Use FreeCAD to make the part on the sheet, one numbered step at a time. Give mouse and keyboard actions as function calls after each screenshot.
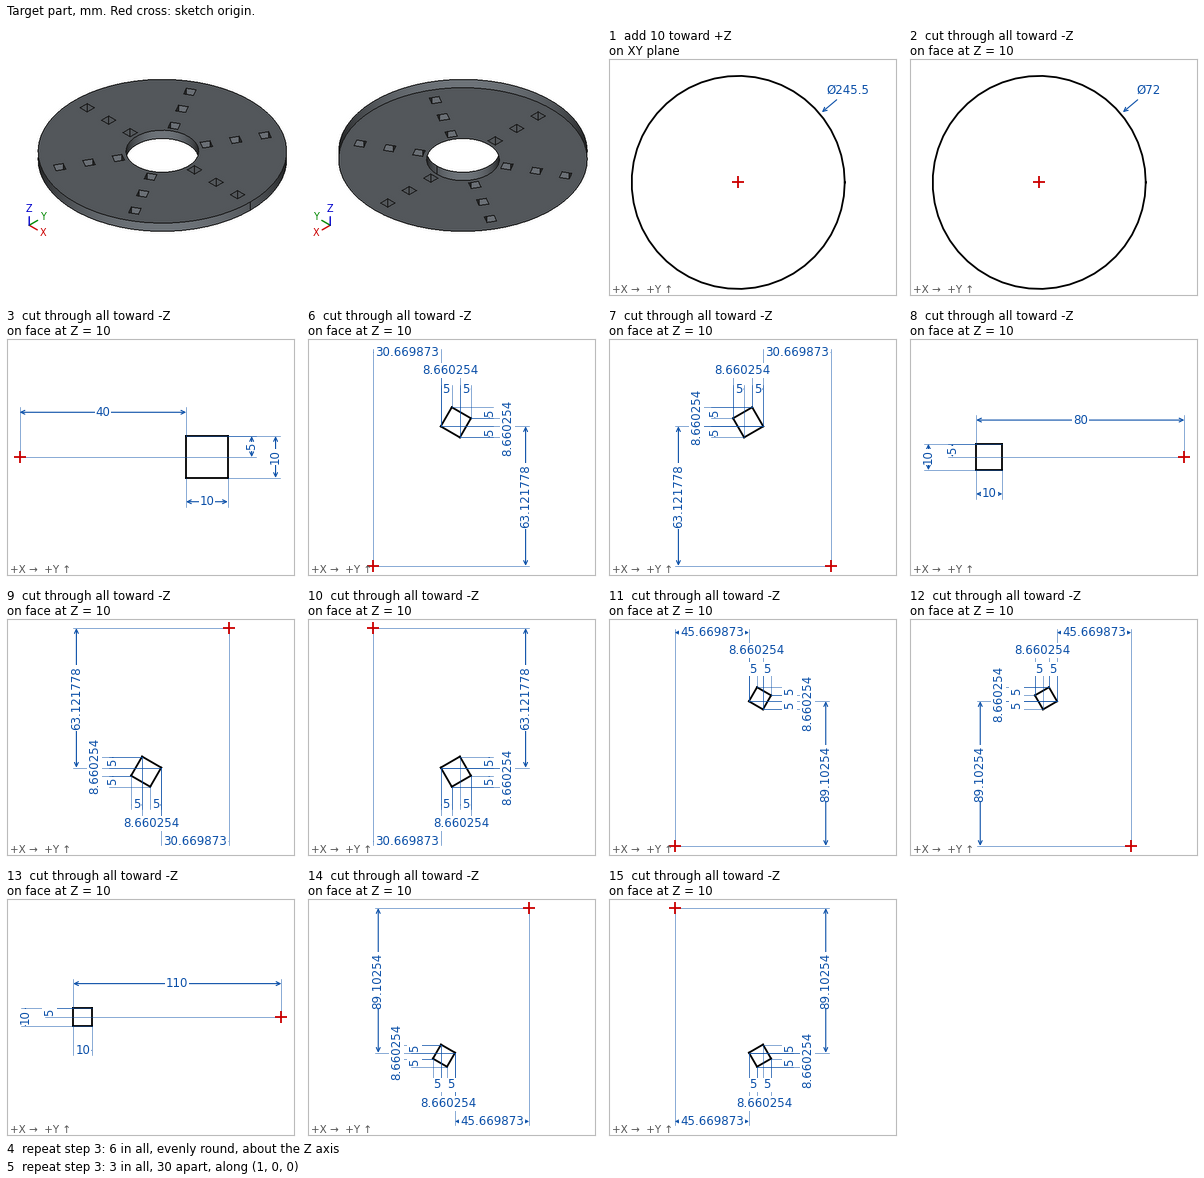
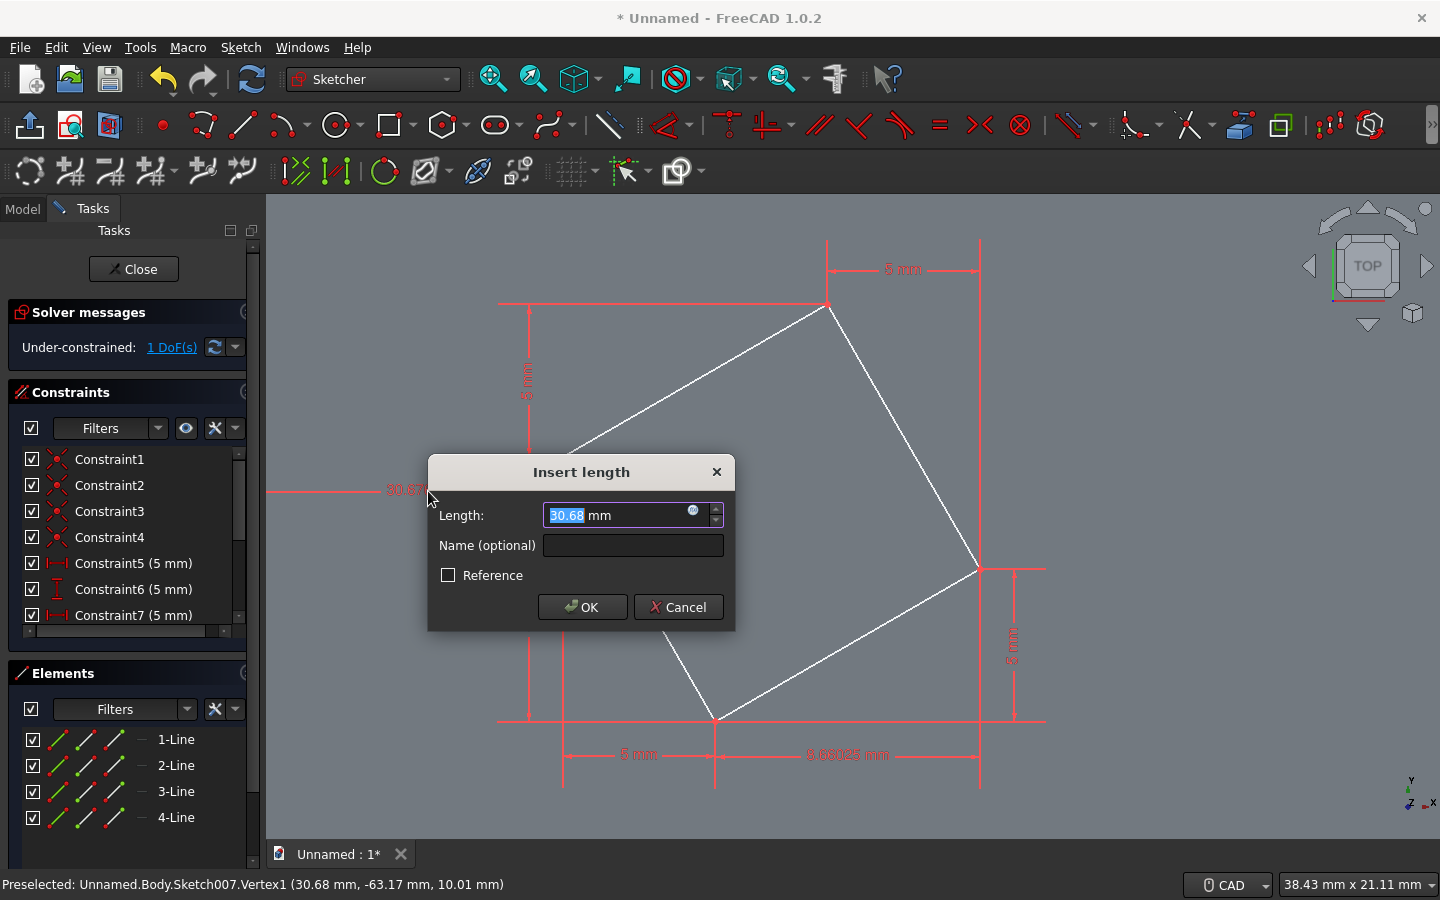
text(30.669873)
key(Return)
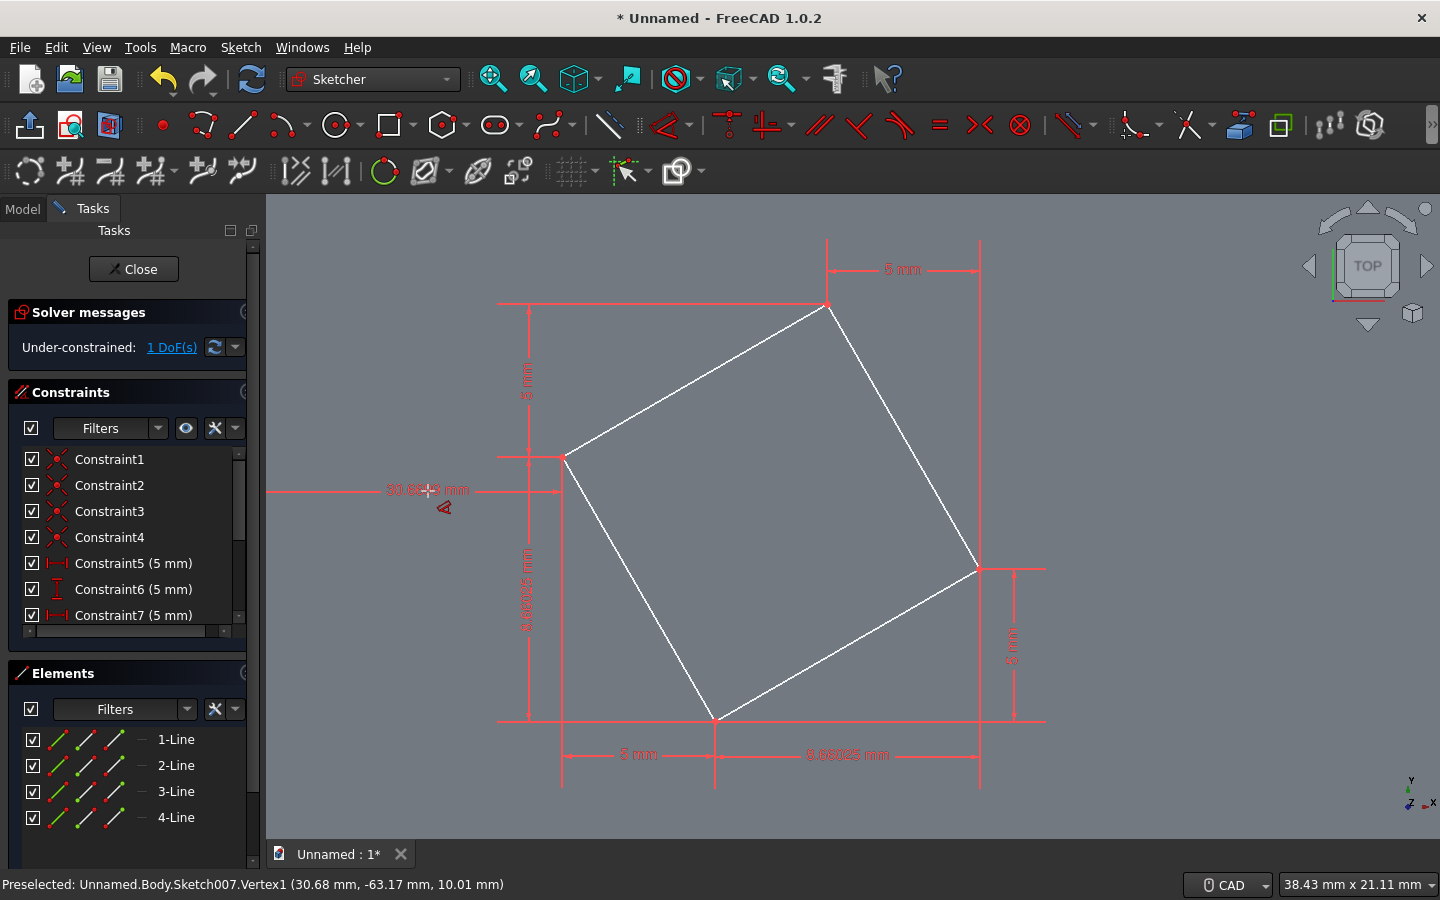
click(562, 457)
click(596, 340)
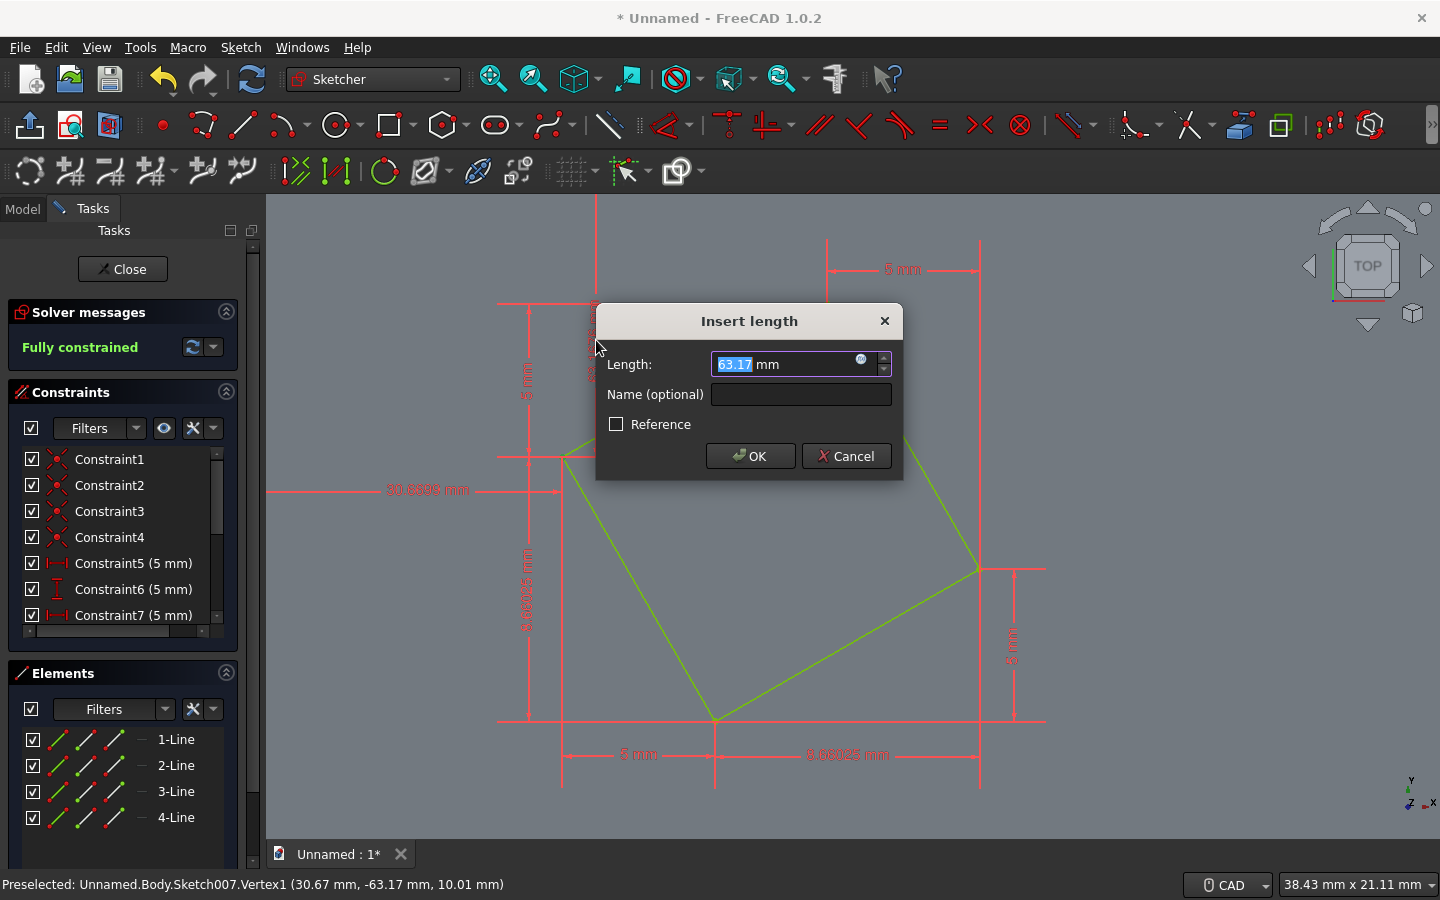
text(63.121778)
key(Return)
key(Escape)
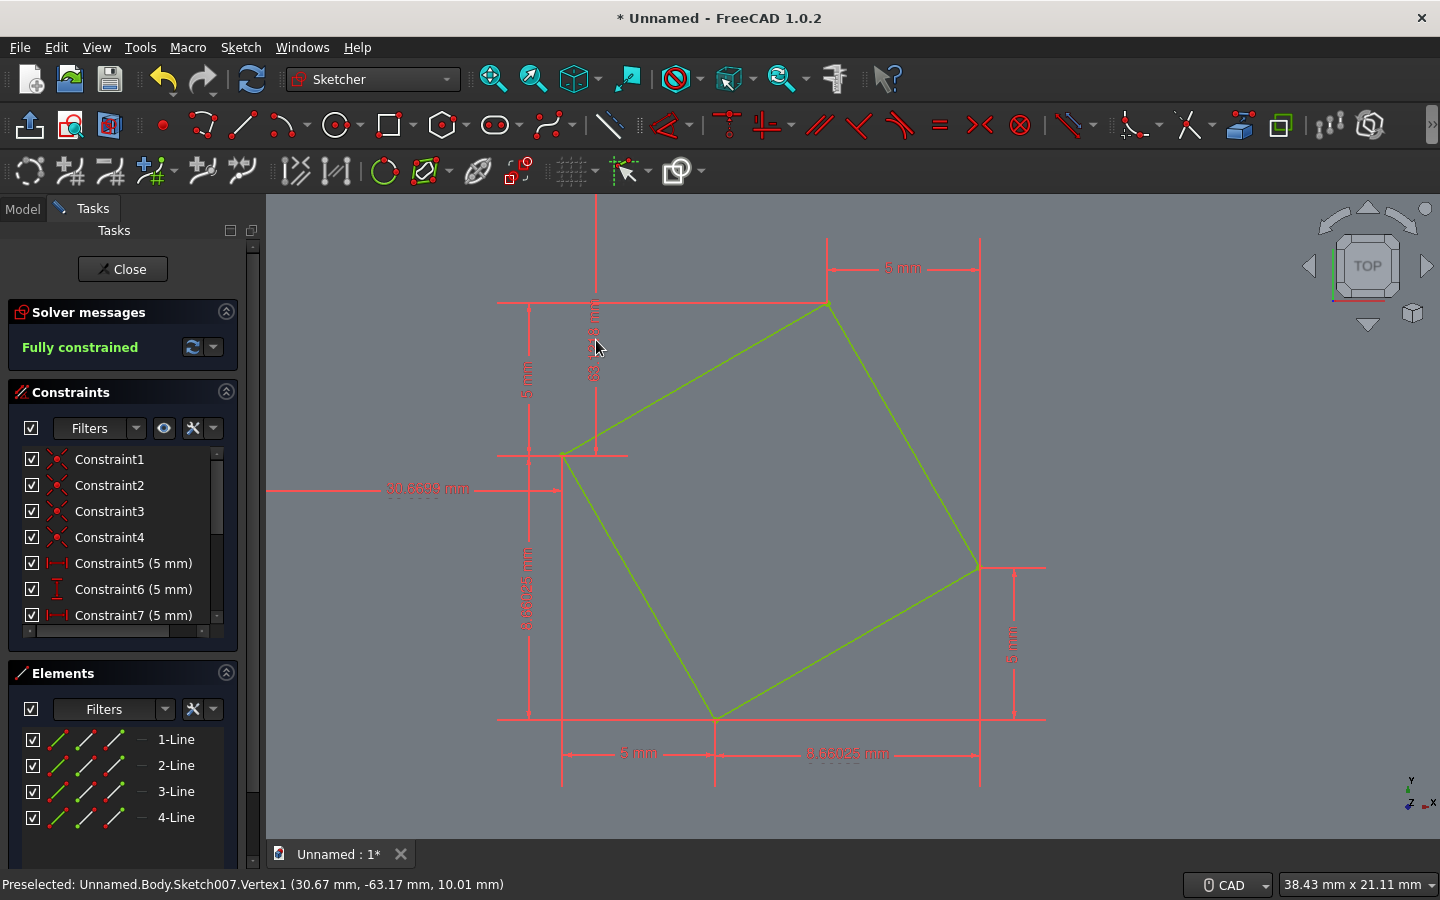
click(123, 269)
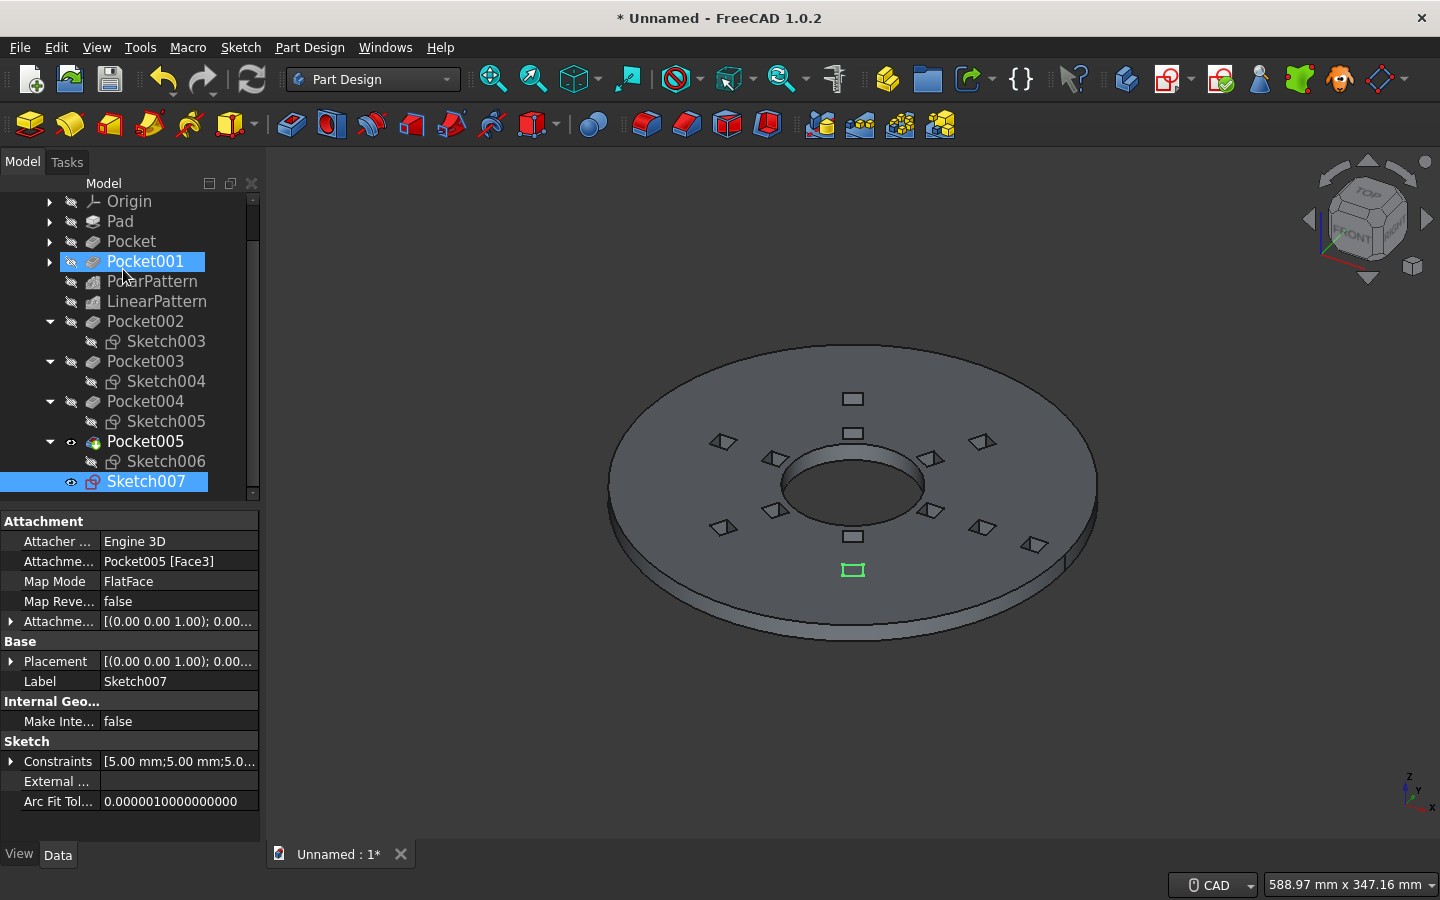
click(292, 124)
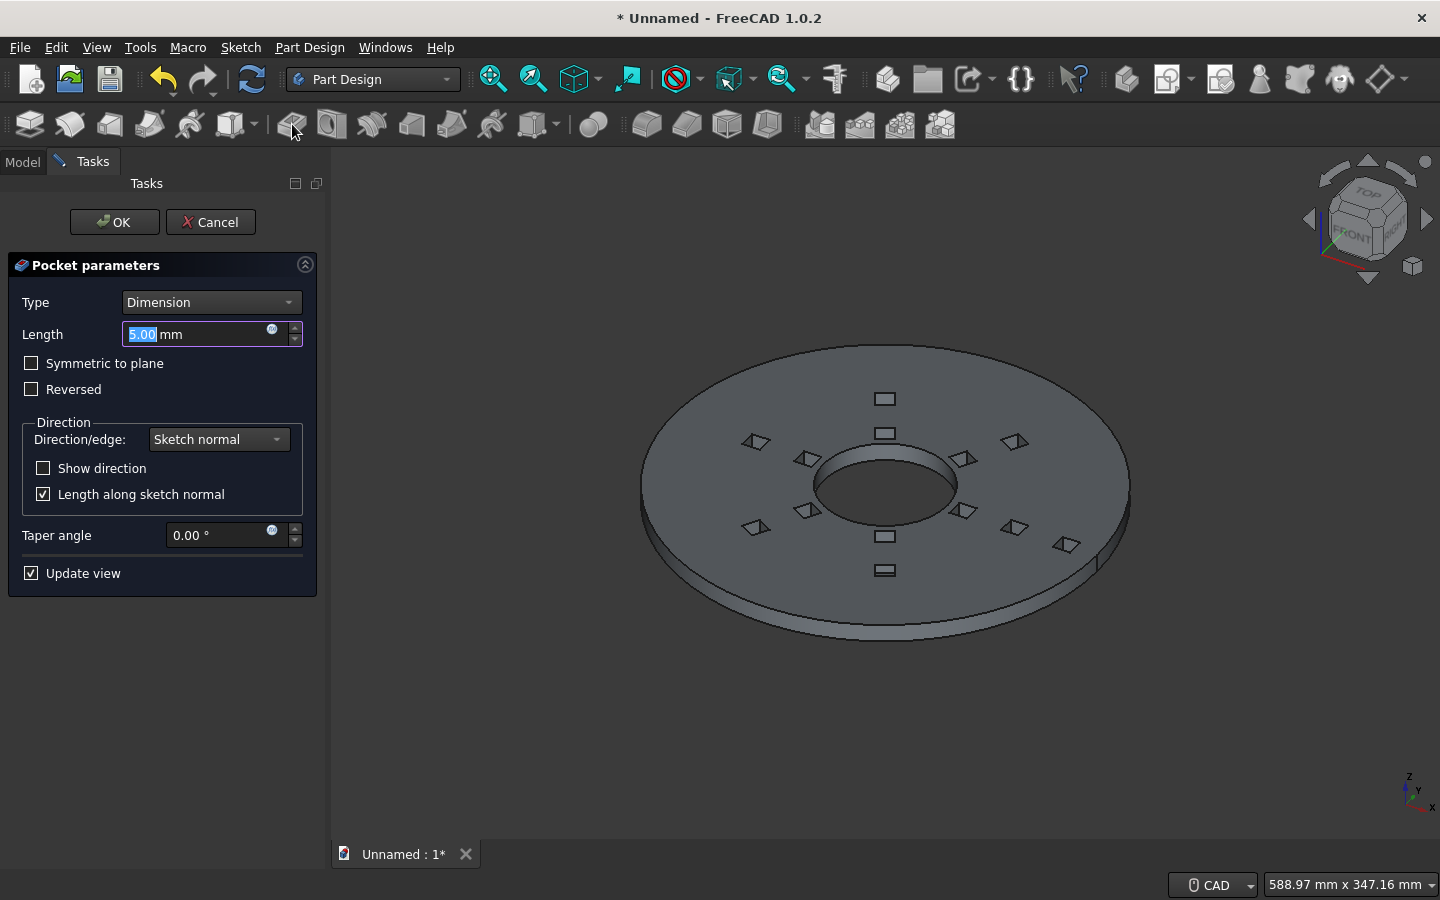
click(212, 302)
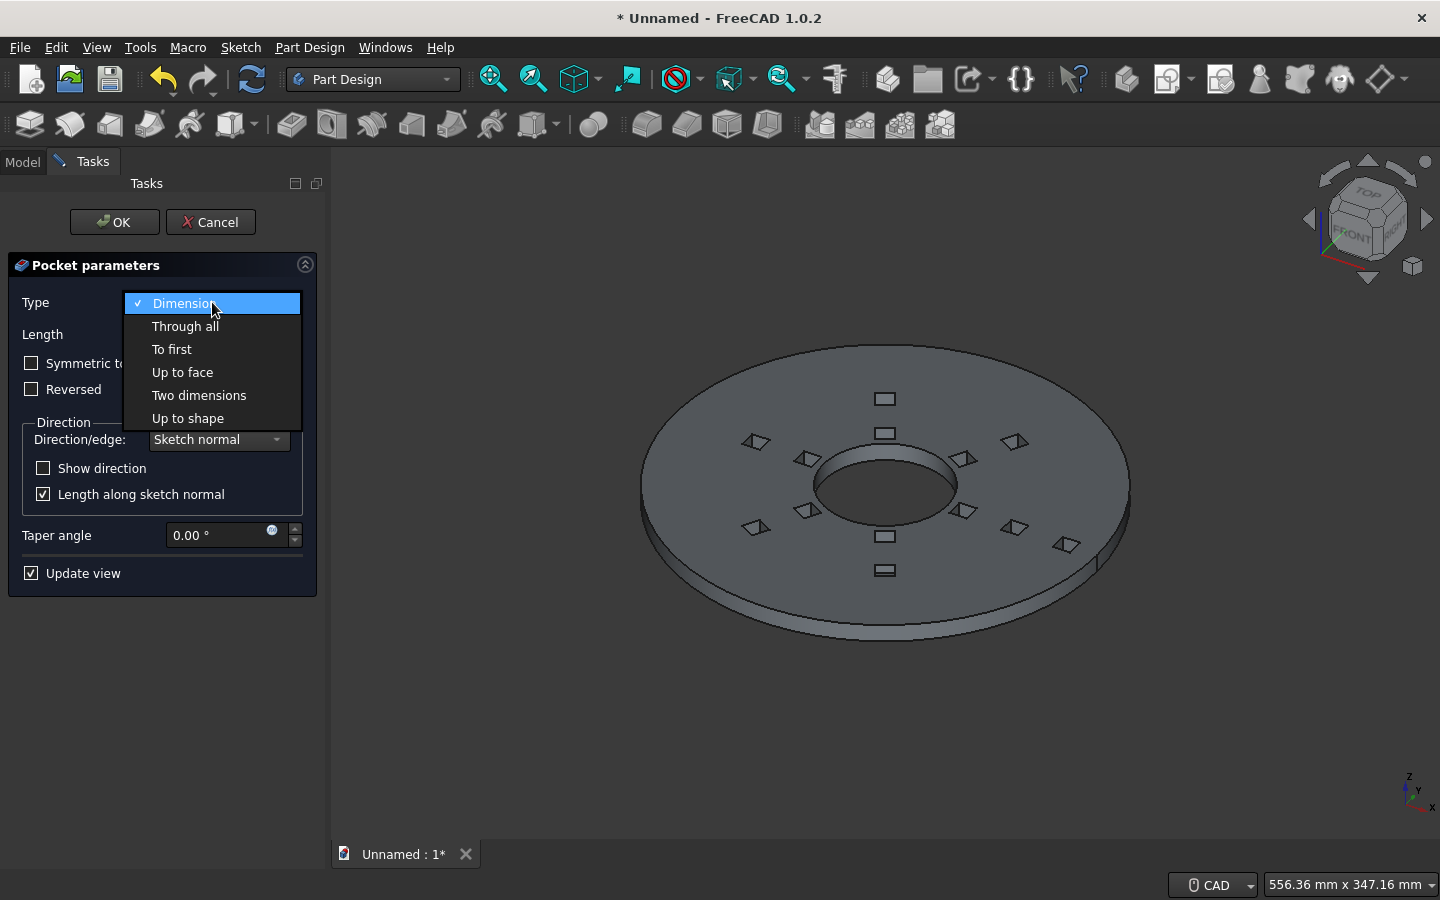
click(212, 326)